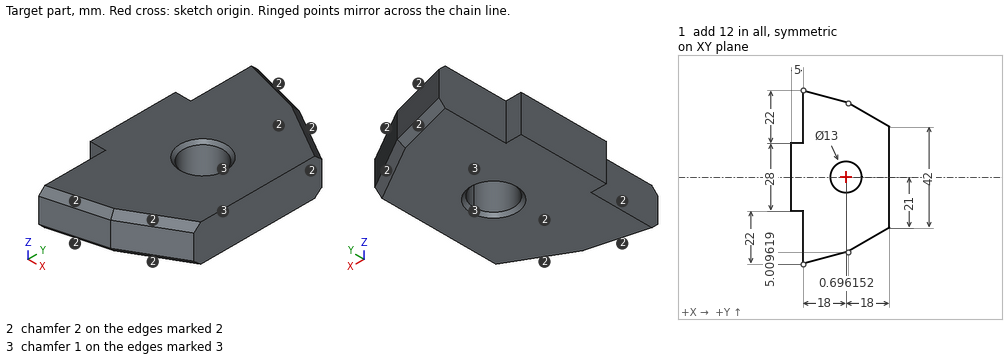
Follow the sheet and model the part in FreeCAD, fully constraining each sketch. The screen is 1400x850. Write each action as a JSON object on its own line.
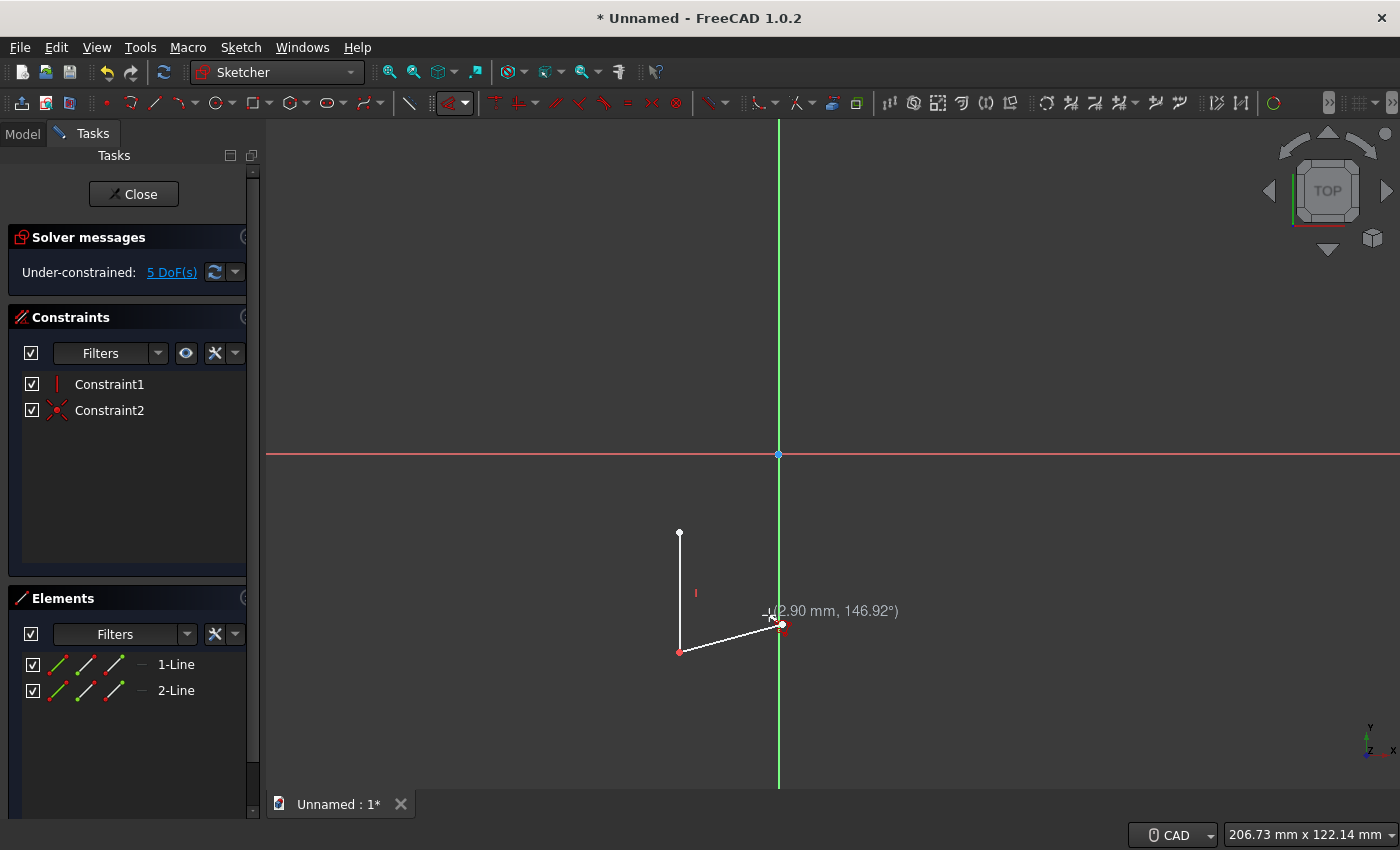
{"action": "left_click", "coordinate": [878, 569]}
{"action": "left_click", "coordinate": [878, 339]}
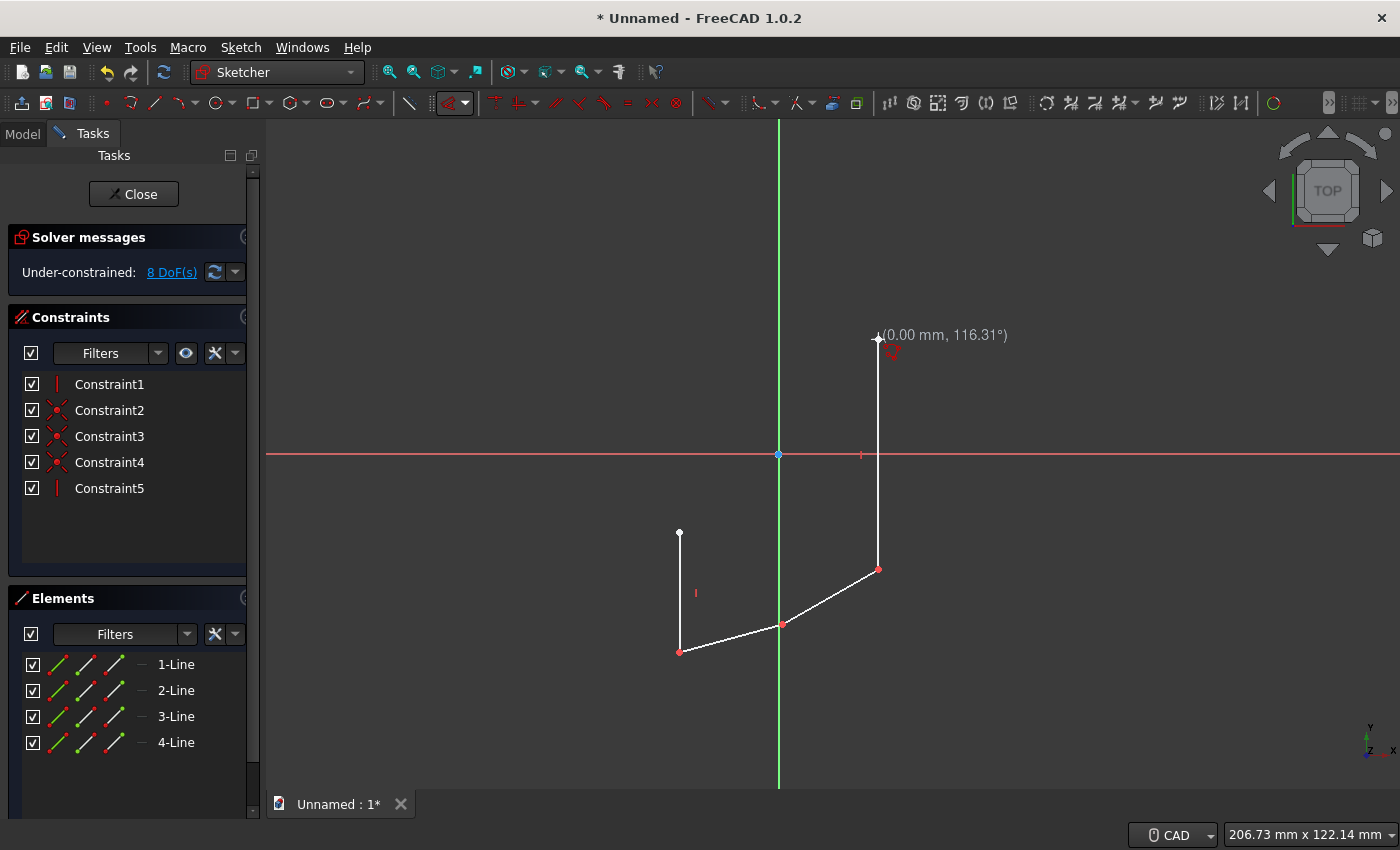
{"action": "scroll", "coordinate": [783, 284], "scroll_direction": "up", "scroll_amount": 8}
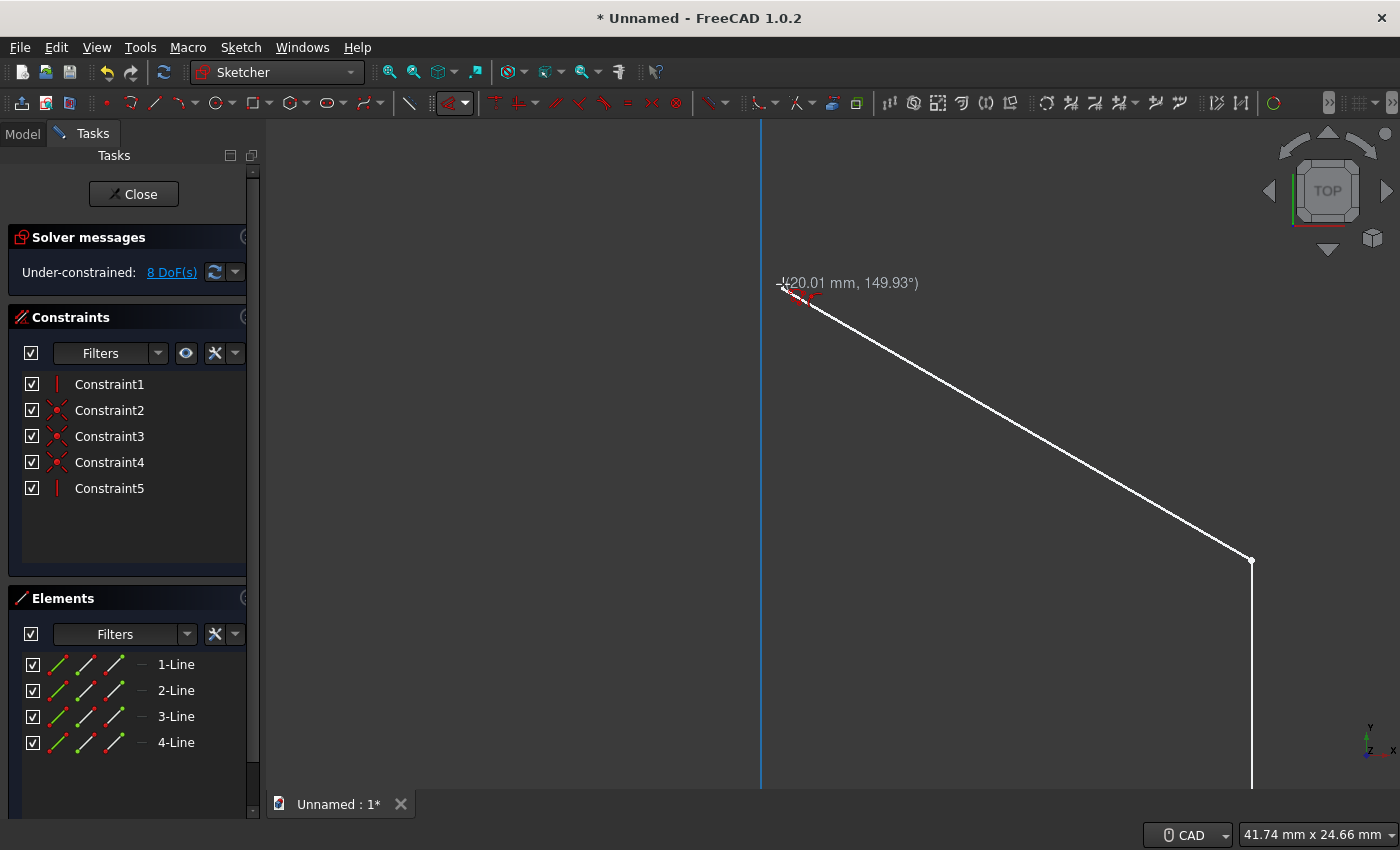
{"action": "left_click", "coordinate": [780, 284]}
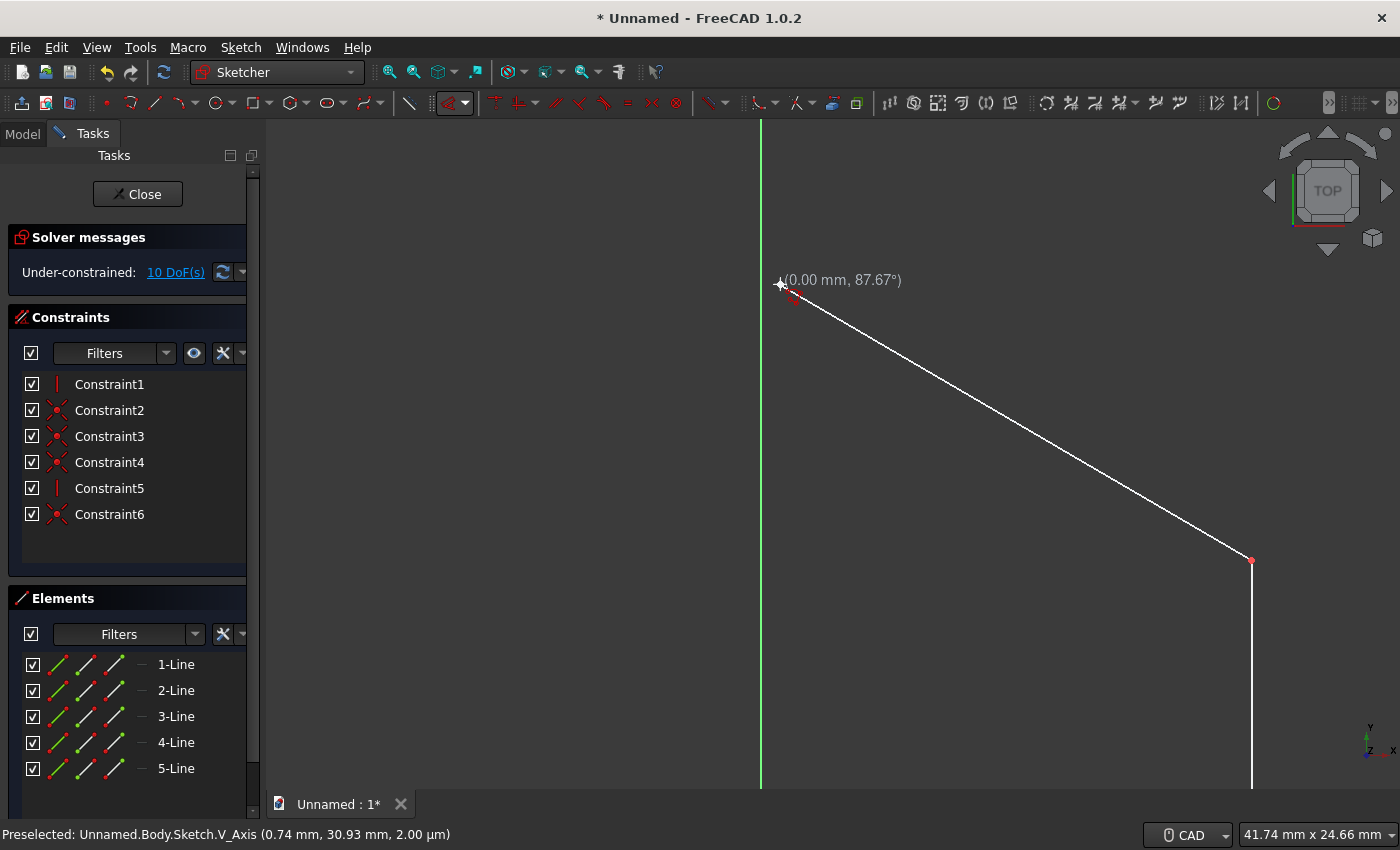
{"action": "scroll", "coordinate": [783, 284], "scroll_direction": "down", "scroll_amount": 8}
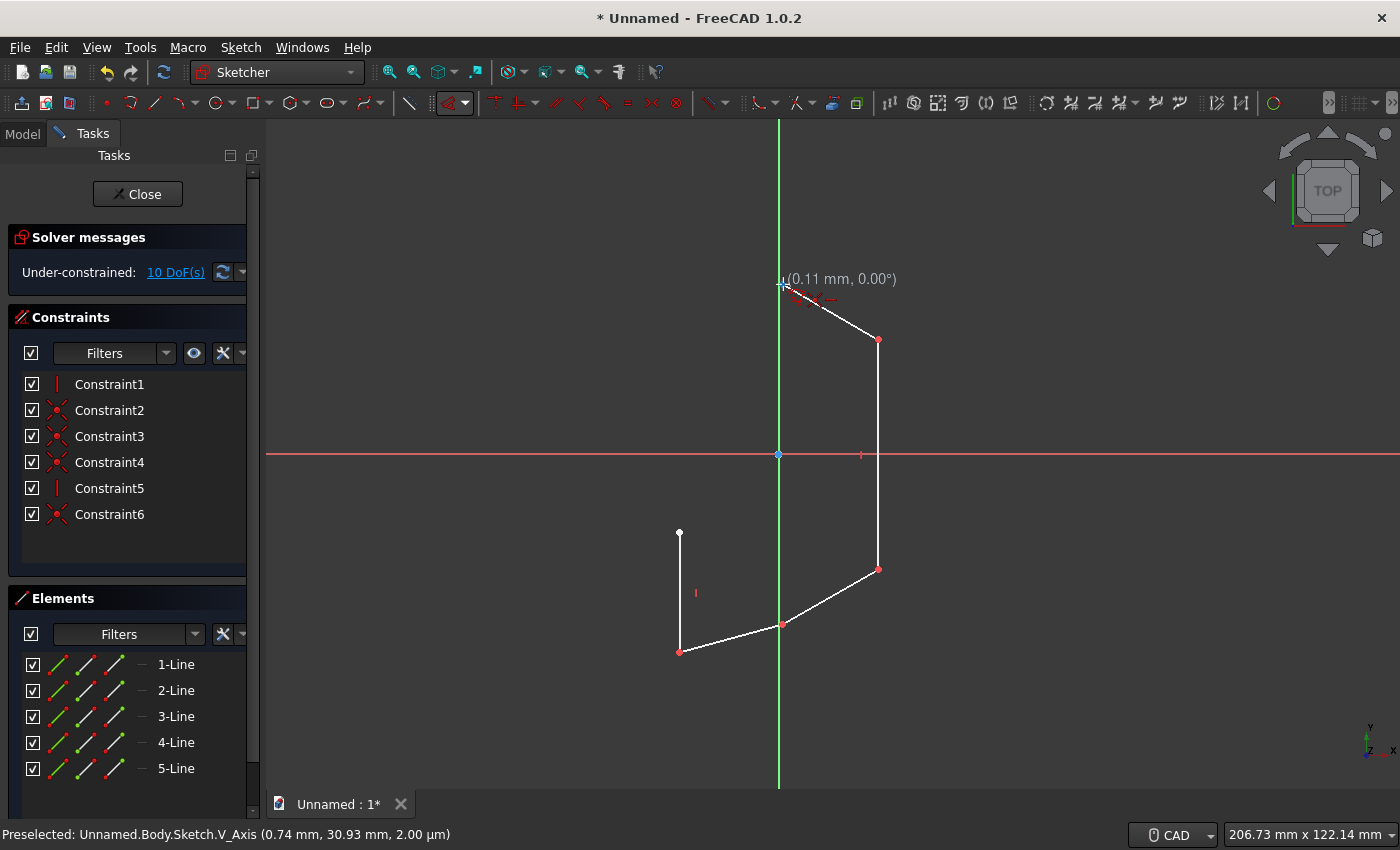
{"action": "left_click", "coordinate": [680, 257]}
{"action": "left_click", "coordinate": [680, 377]}
{"action": "left_click", "coordinate": [653, 377]}
{"action": "left_click", "coordinate": [653, 531]}
{"action": "left_click", "coordinate": [680, 532]}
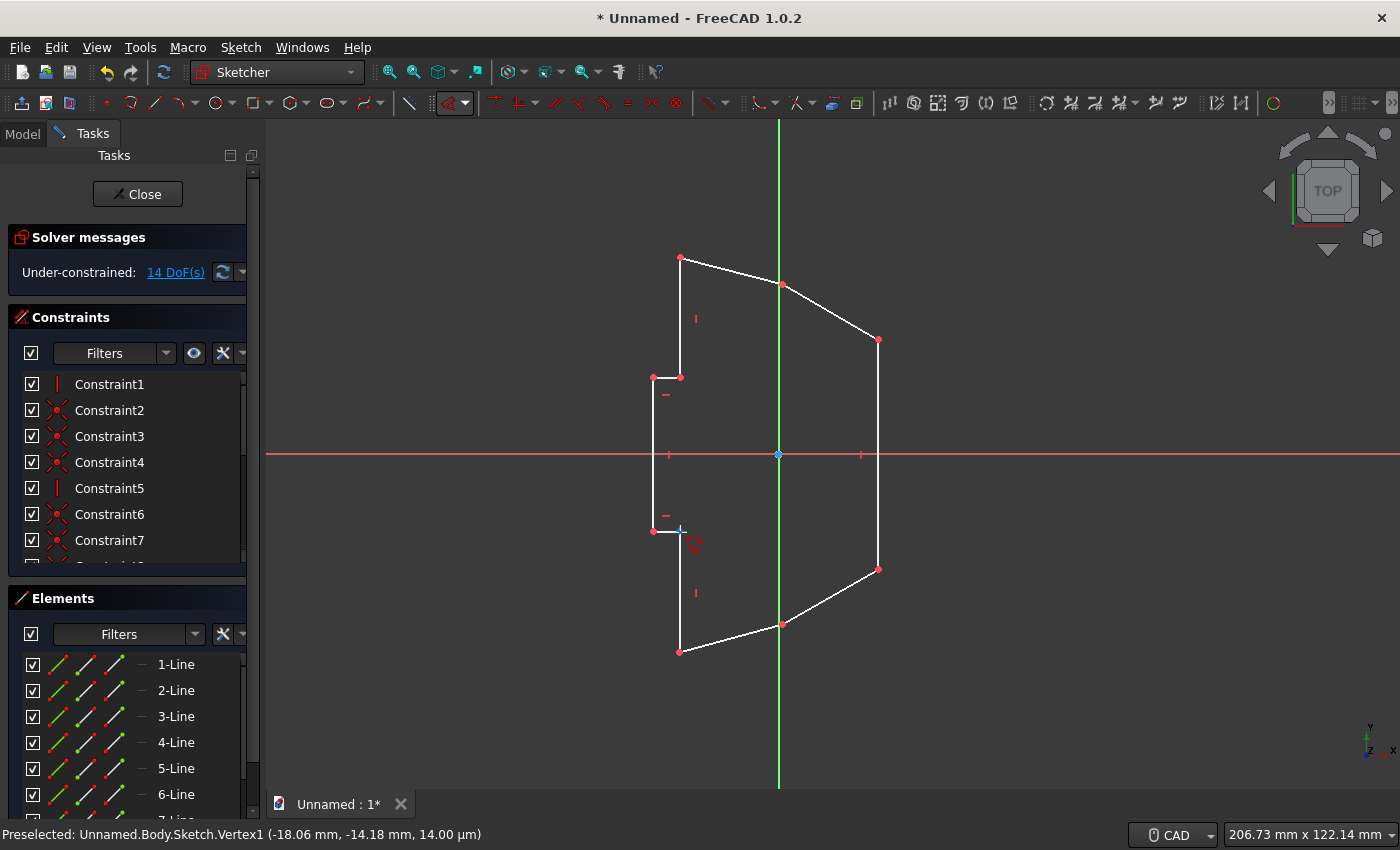
{"action": "left_click", "coordinate": [216, 104]}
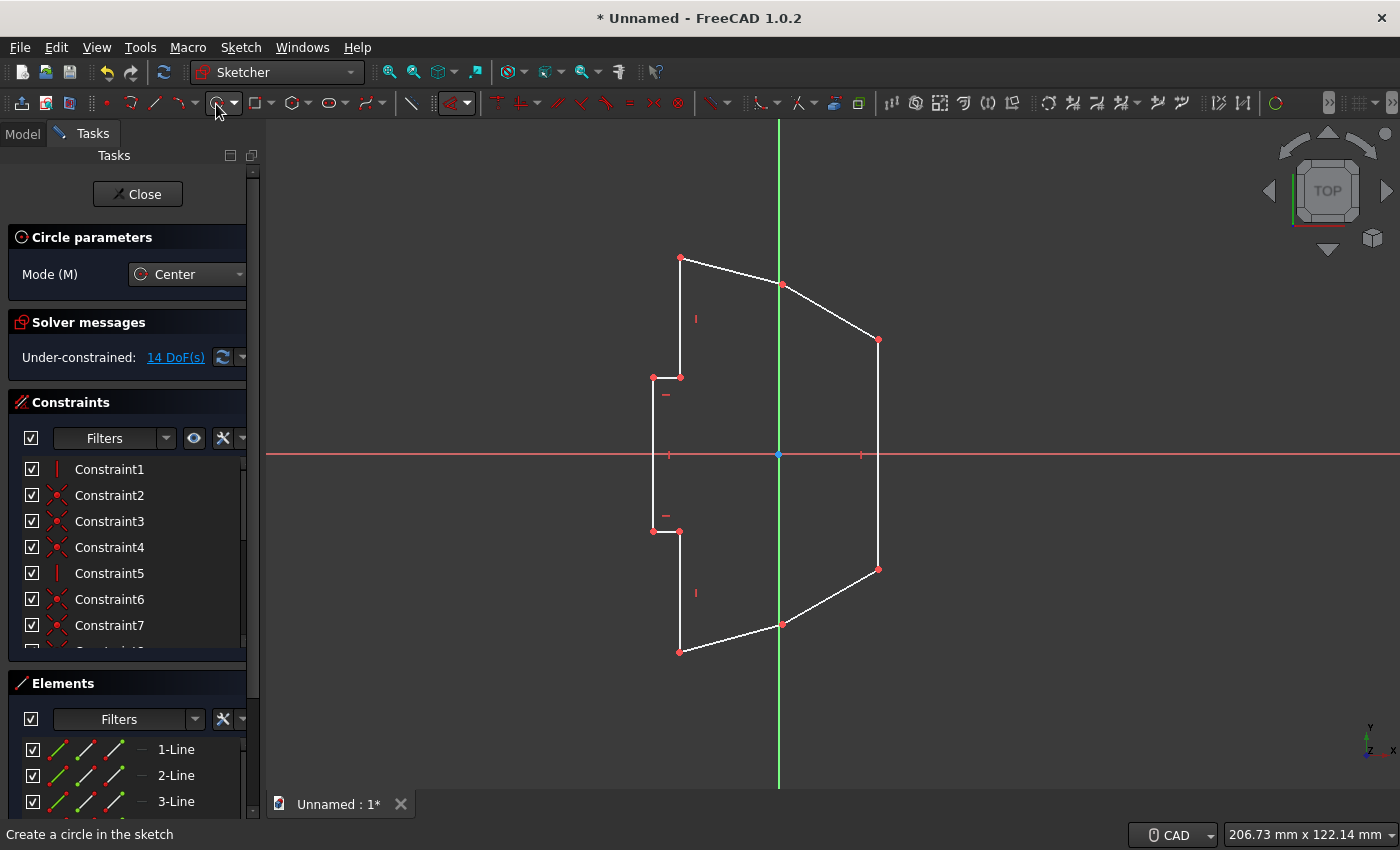
{"action": "left_click", "coordinate": [779, 454]}
{"action": "left_click", "coordinate": [804, 429]}
{"action": "key", "text": "Escape"}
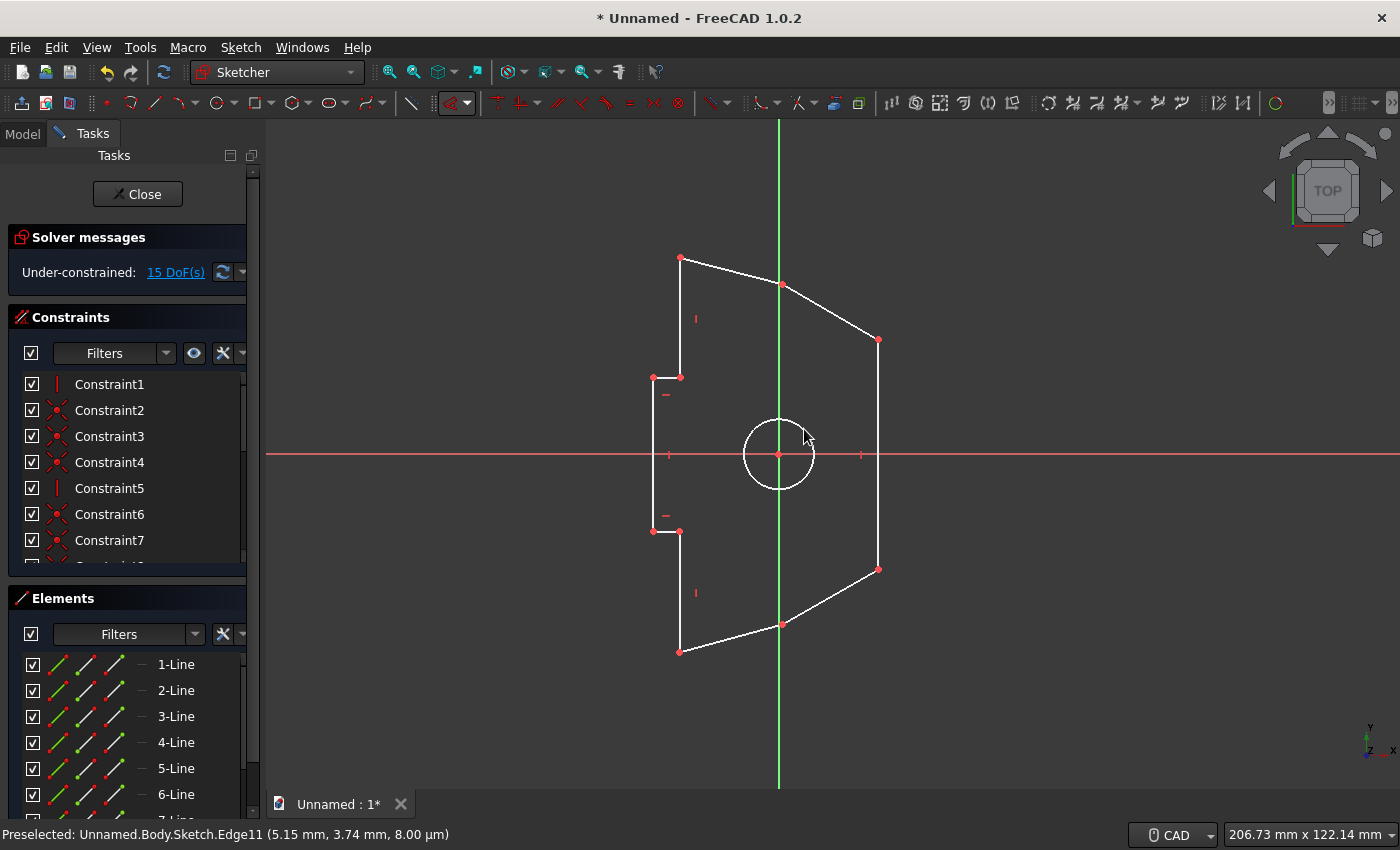
{"action": "left_click", "coordinate": [783, 624]}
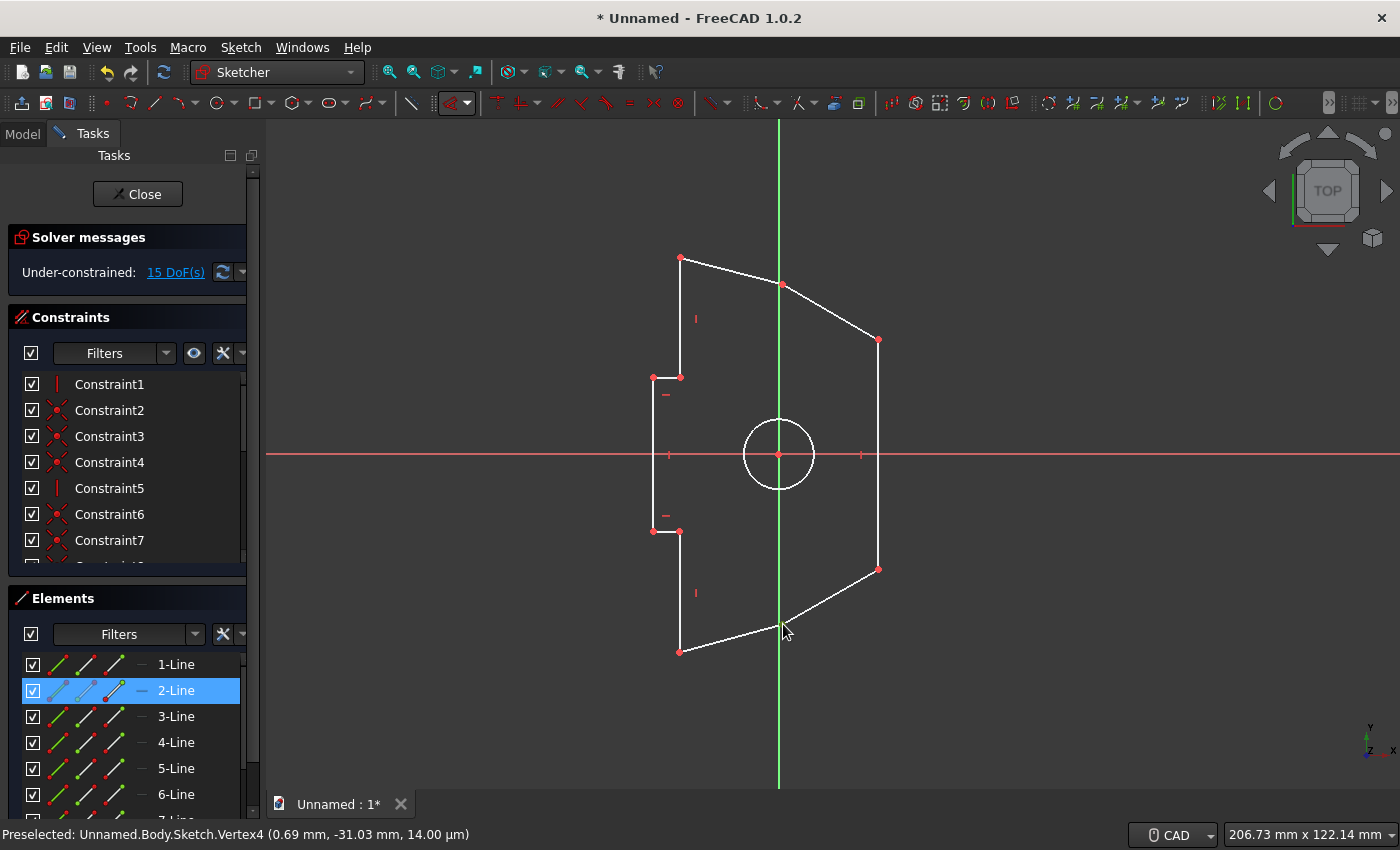
{"action": "left_click", "coordinate": [783, 284]}